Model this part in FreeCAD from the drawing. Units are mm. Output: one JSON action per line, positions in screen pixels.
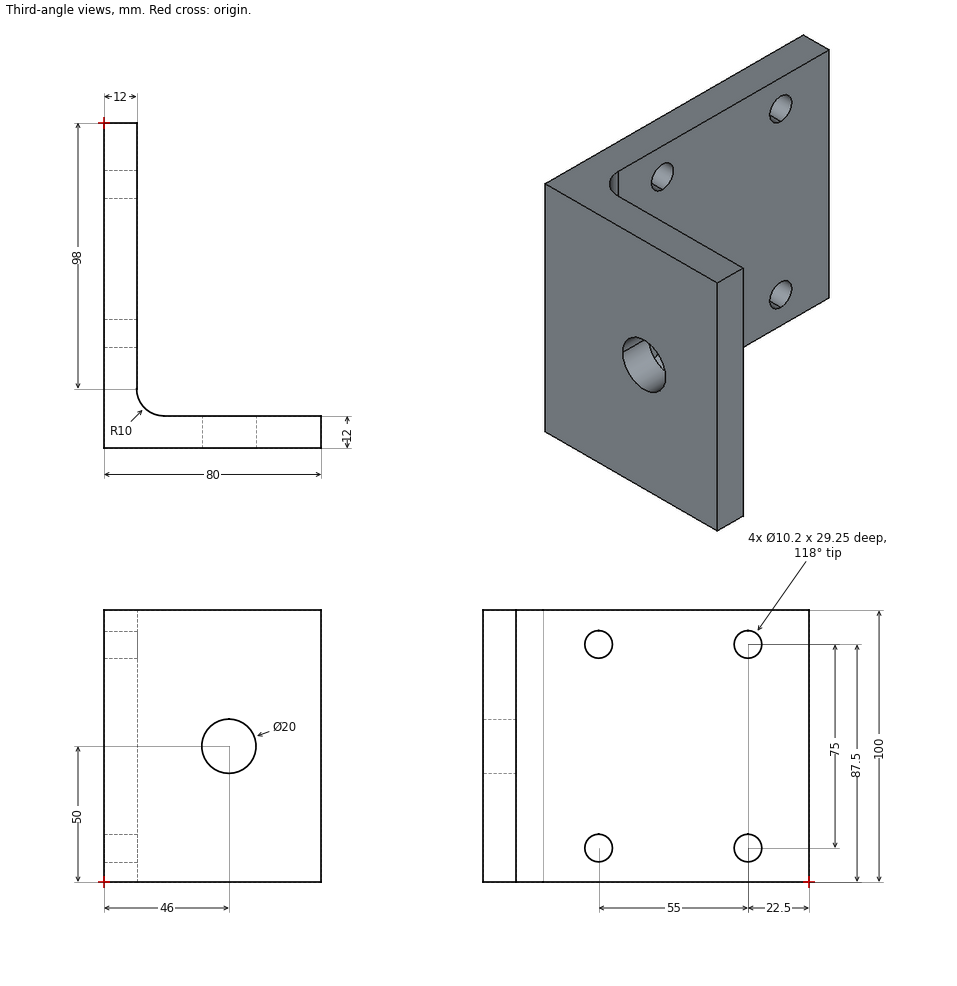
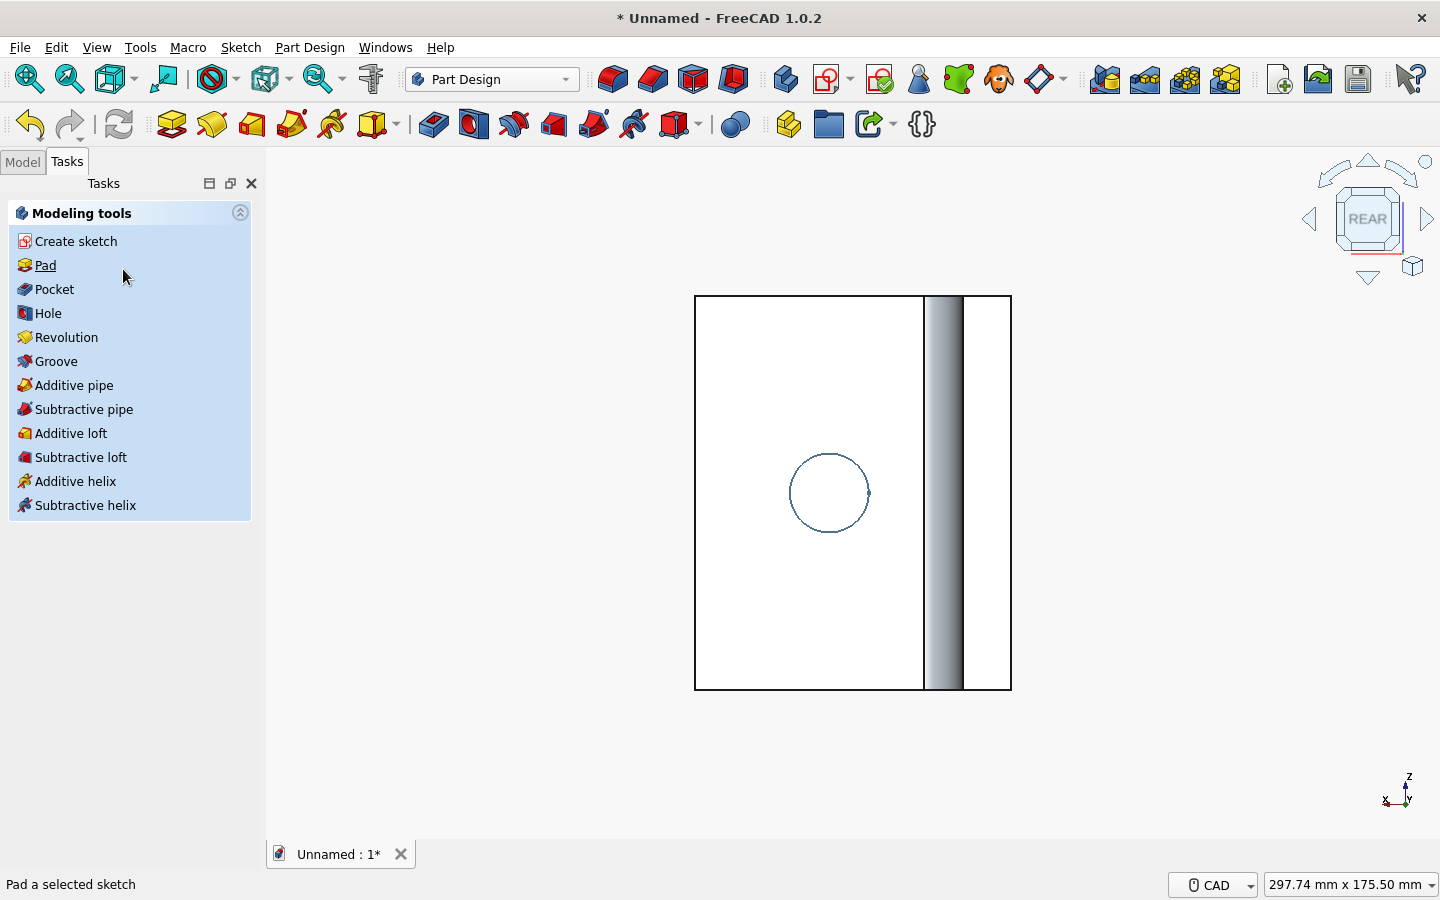
{"action": "left_click", "coordinate": [434, 124]}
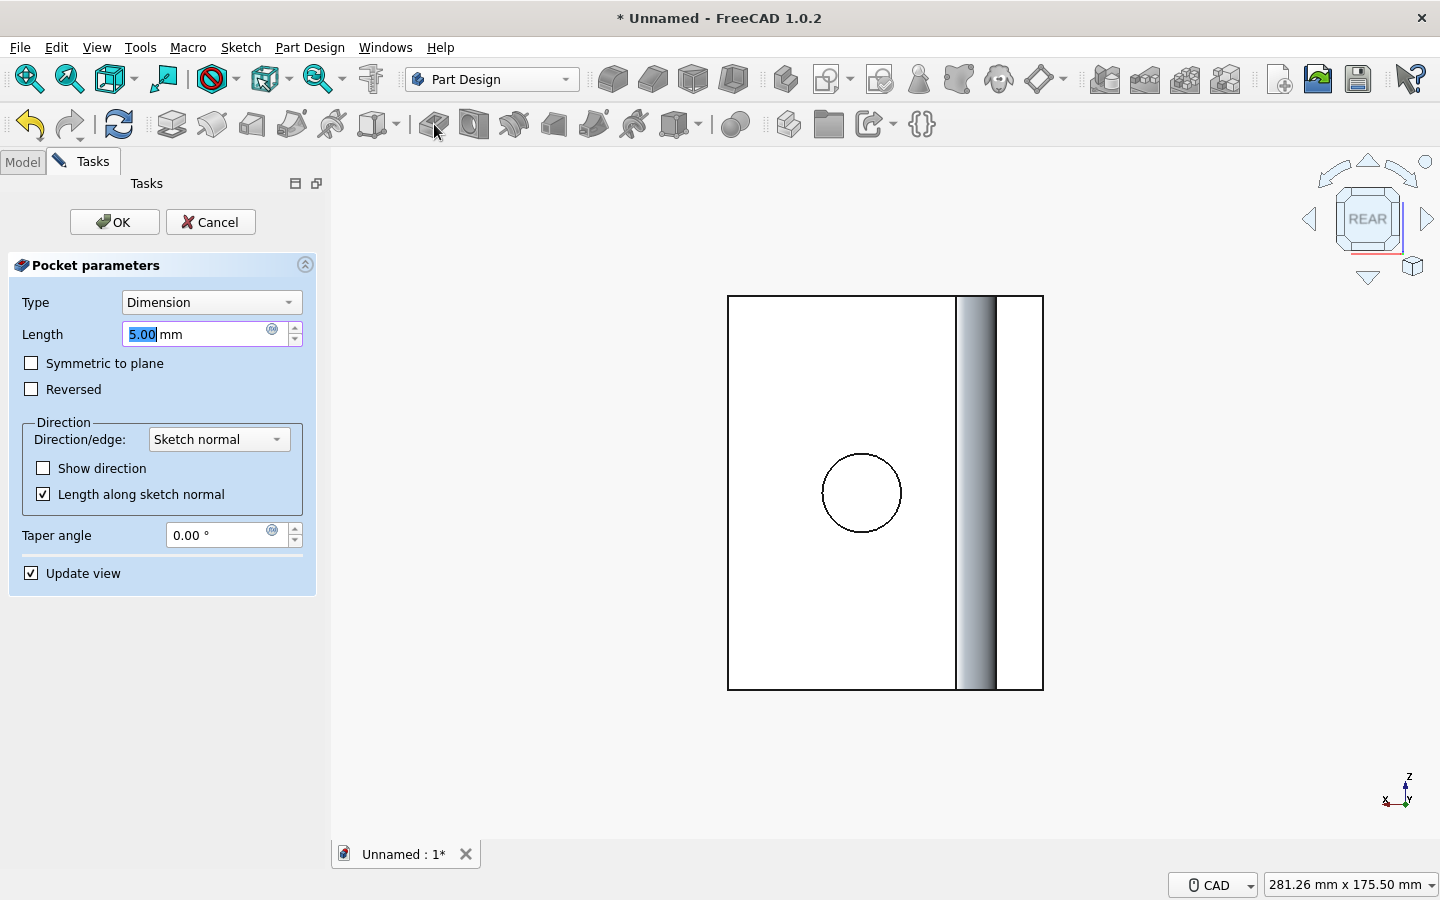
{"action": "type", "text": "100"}
{"action": "key", "text": "Tab"}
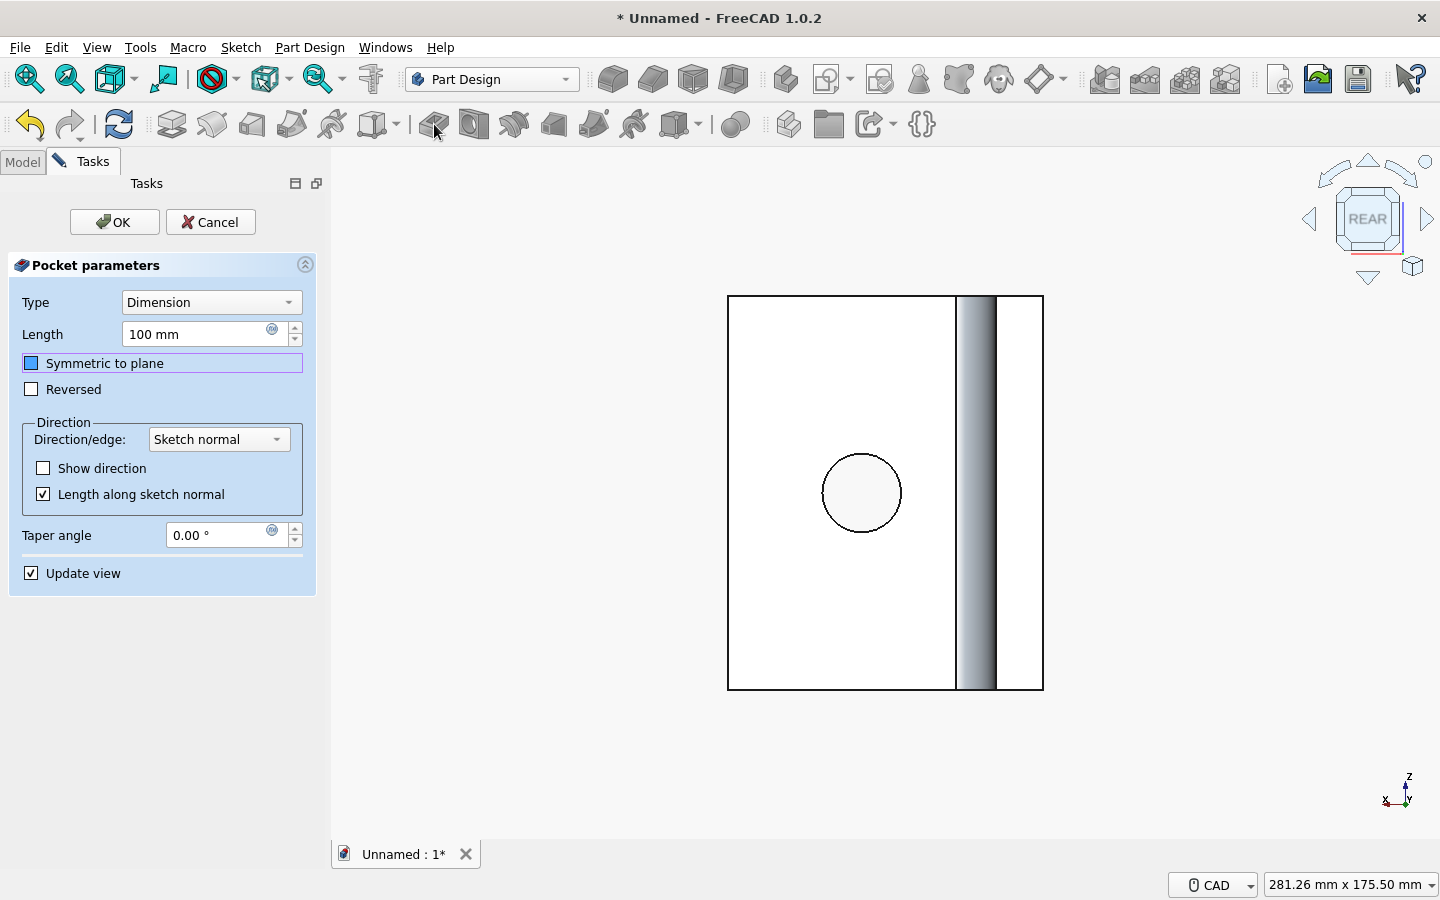
{"action": "left_click", "coordinate": [115, 222]}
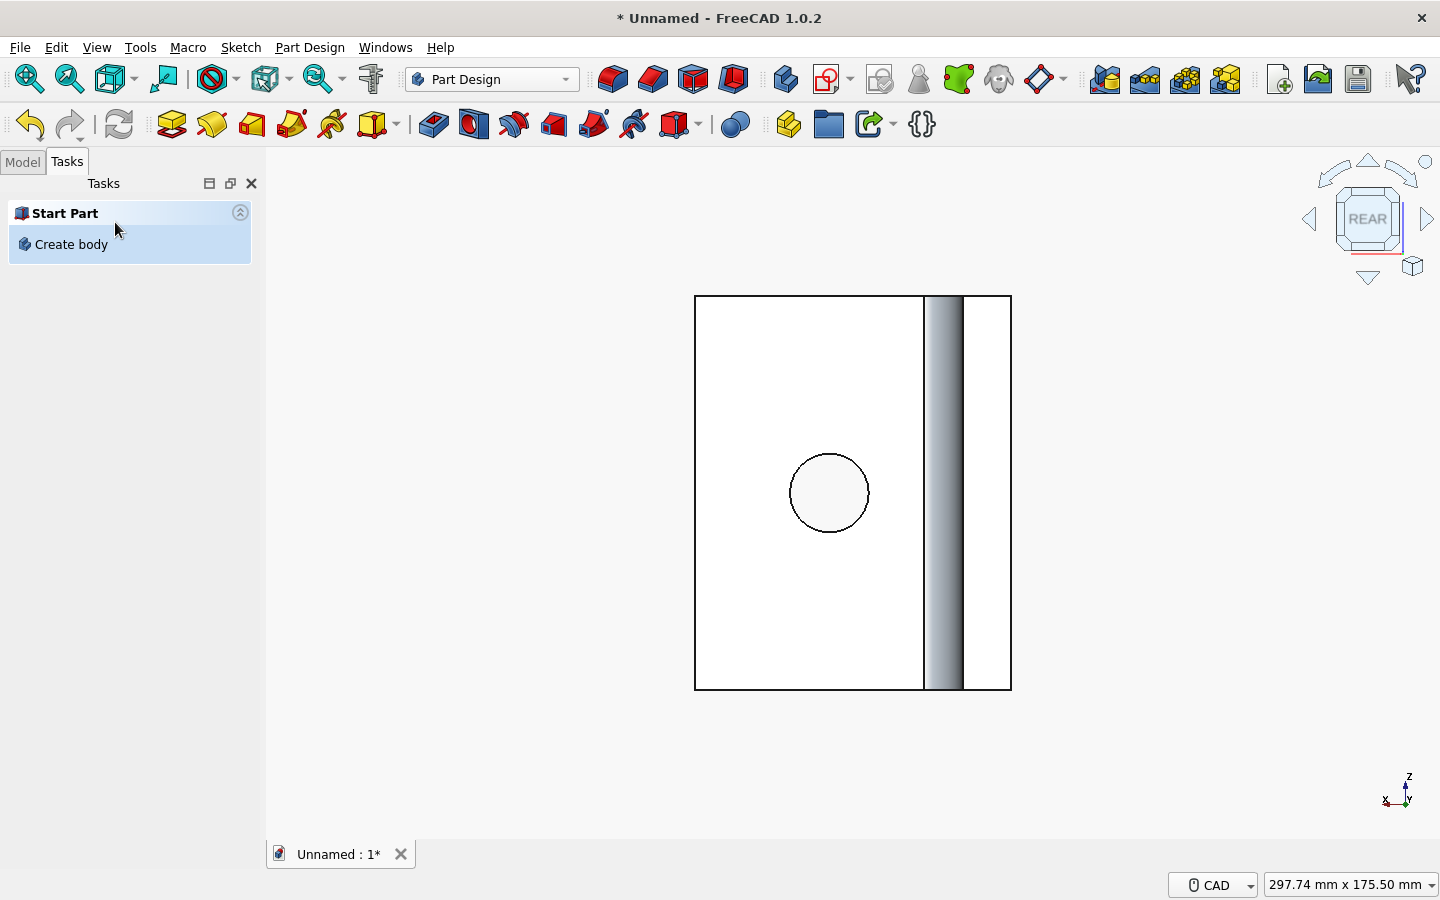
{"action": "key", "text": "0"}